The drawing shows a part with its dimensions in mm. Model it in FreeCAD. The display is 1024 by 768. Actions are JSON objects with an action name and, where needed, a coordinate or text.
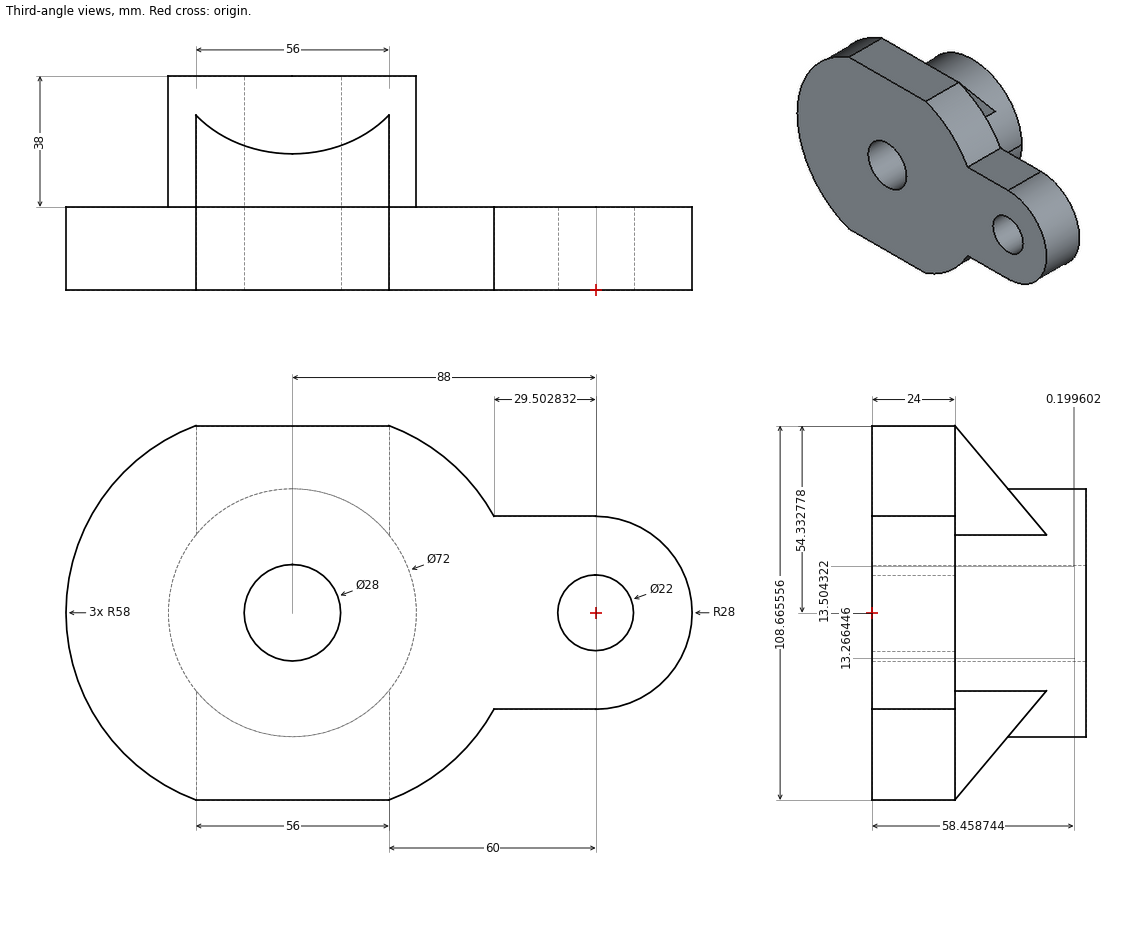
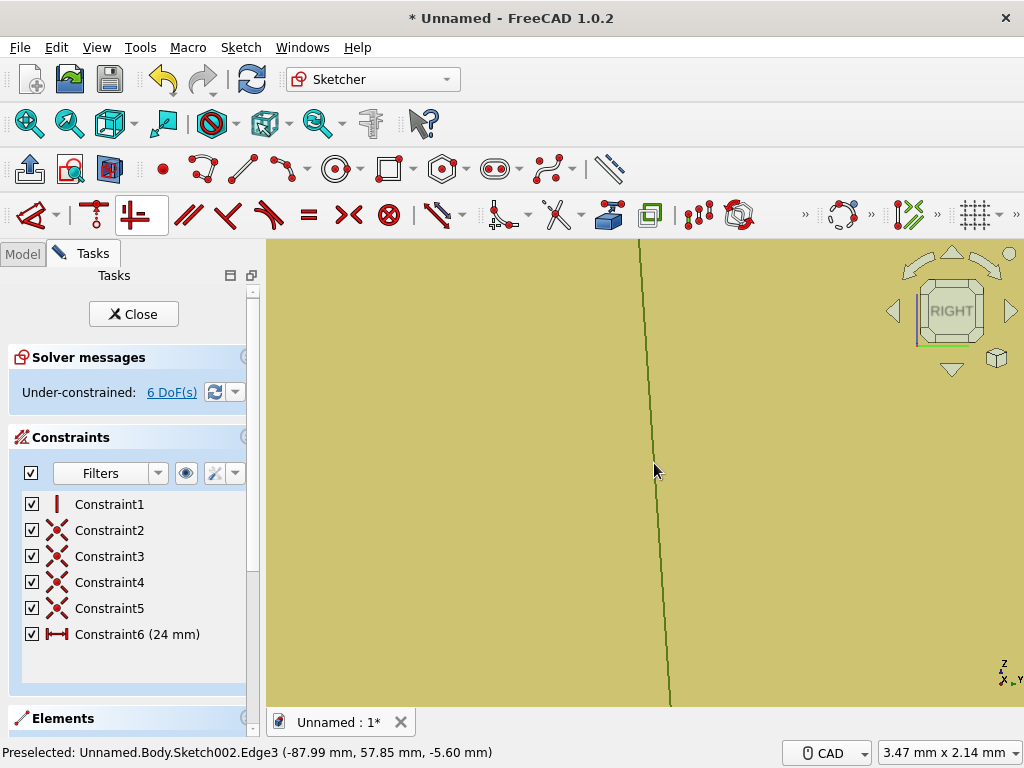
{"action": "left_click", "coordinate": [58, 216]}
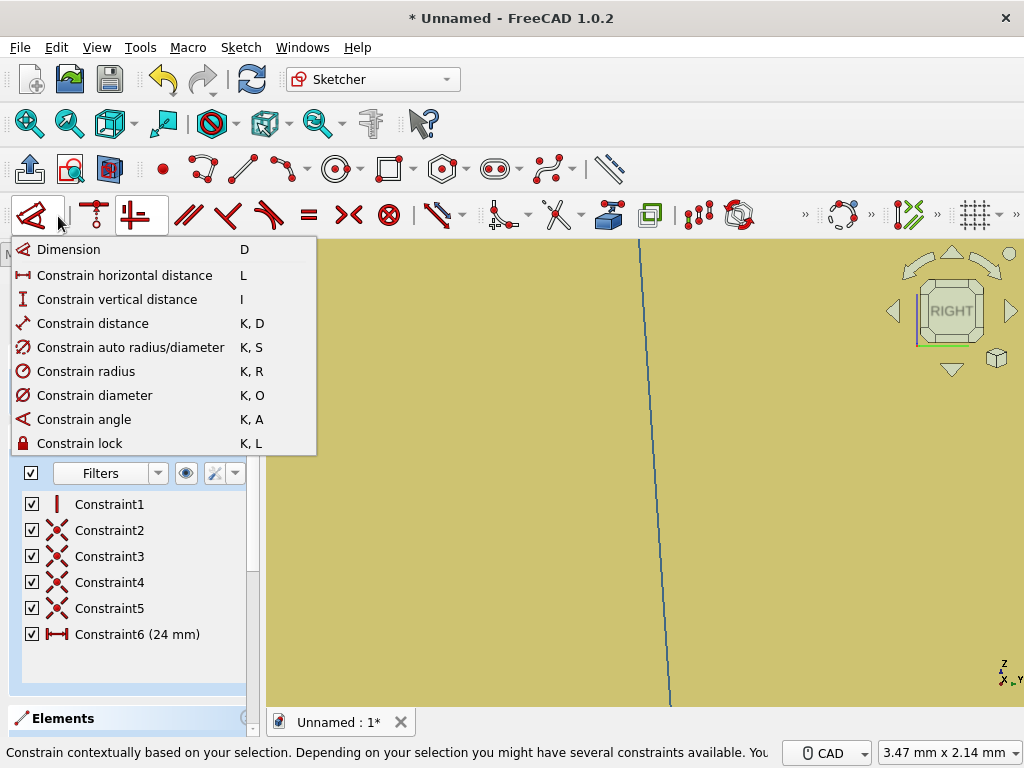
{"action": "left_click", "coordinate": [164, 275]}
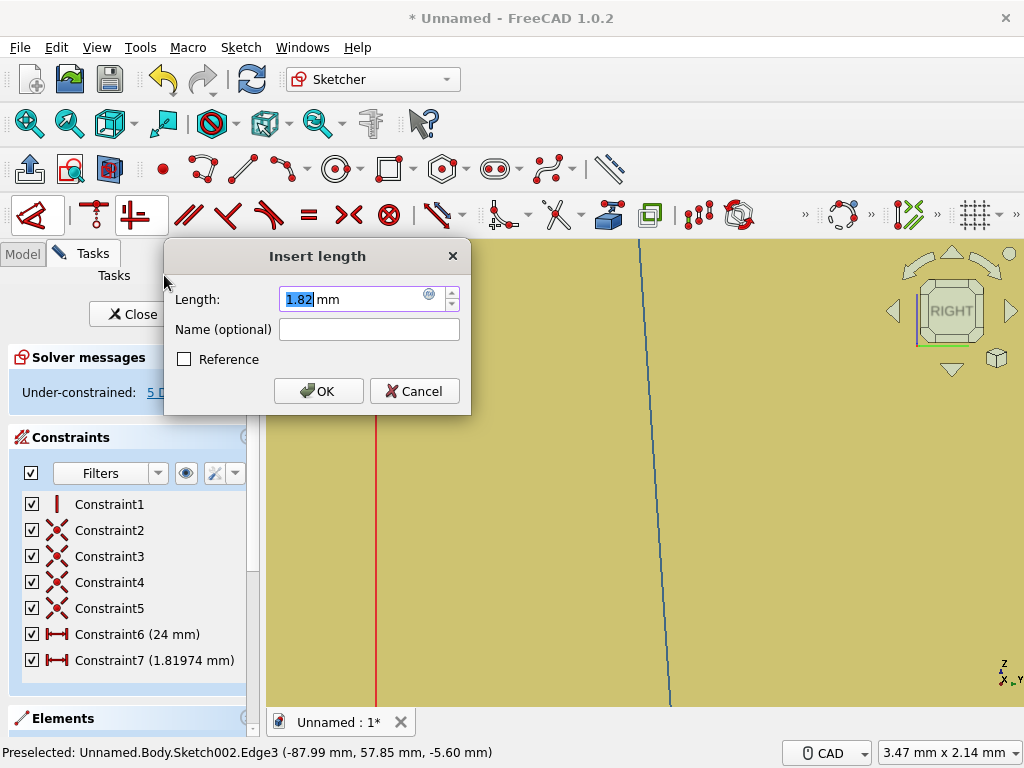
{"action": "type", "text": "0.199602"}
{"action": "key", "text": "Return"}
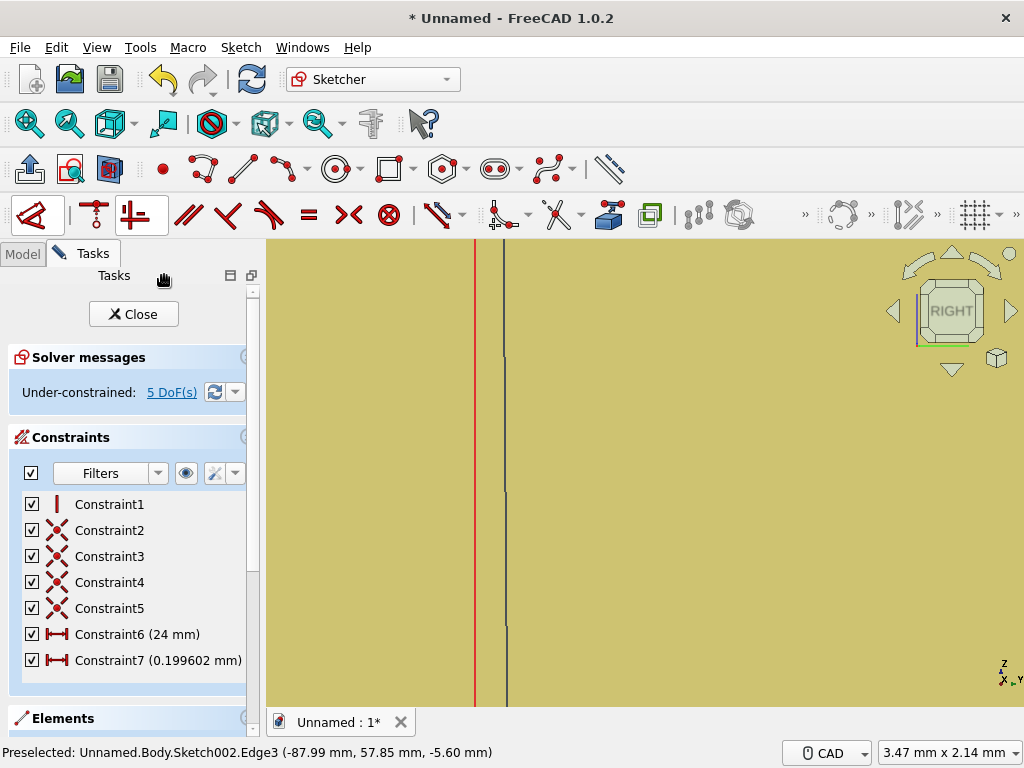
{"action": "scroll", "coordinate": [576, 473], "scroll_direction": "down", "scroll_amount": 15}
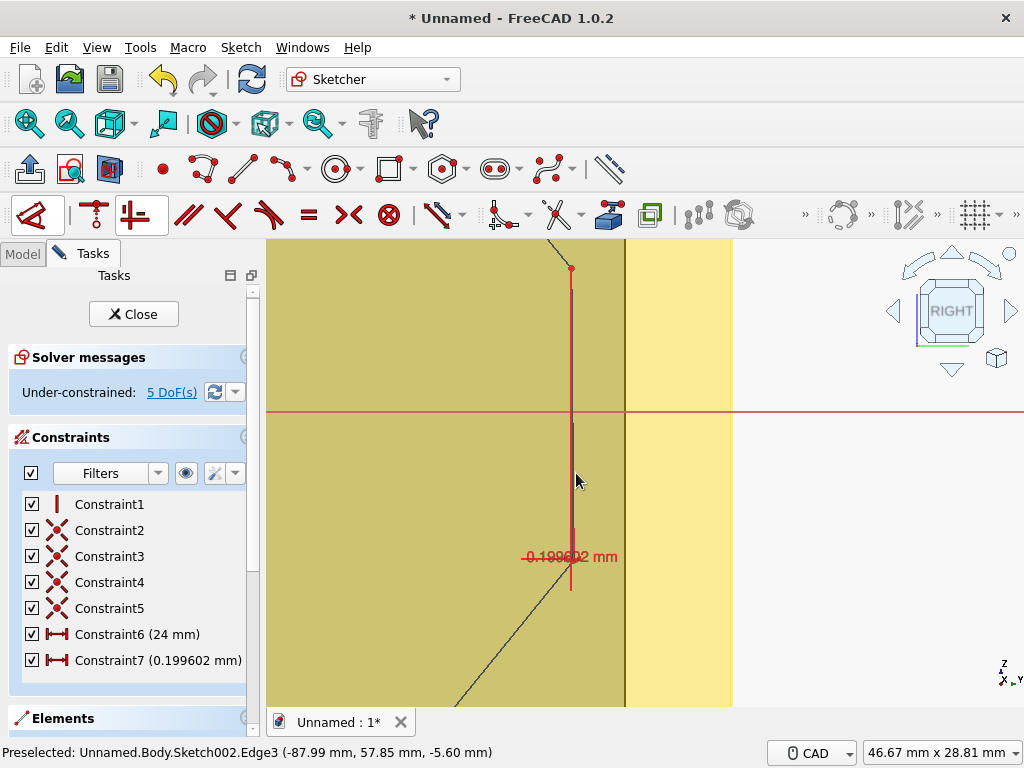
{"action": "scroll", "coordinate": [677, 493], "scroll_direction": "down", "scroll_amount": 7}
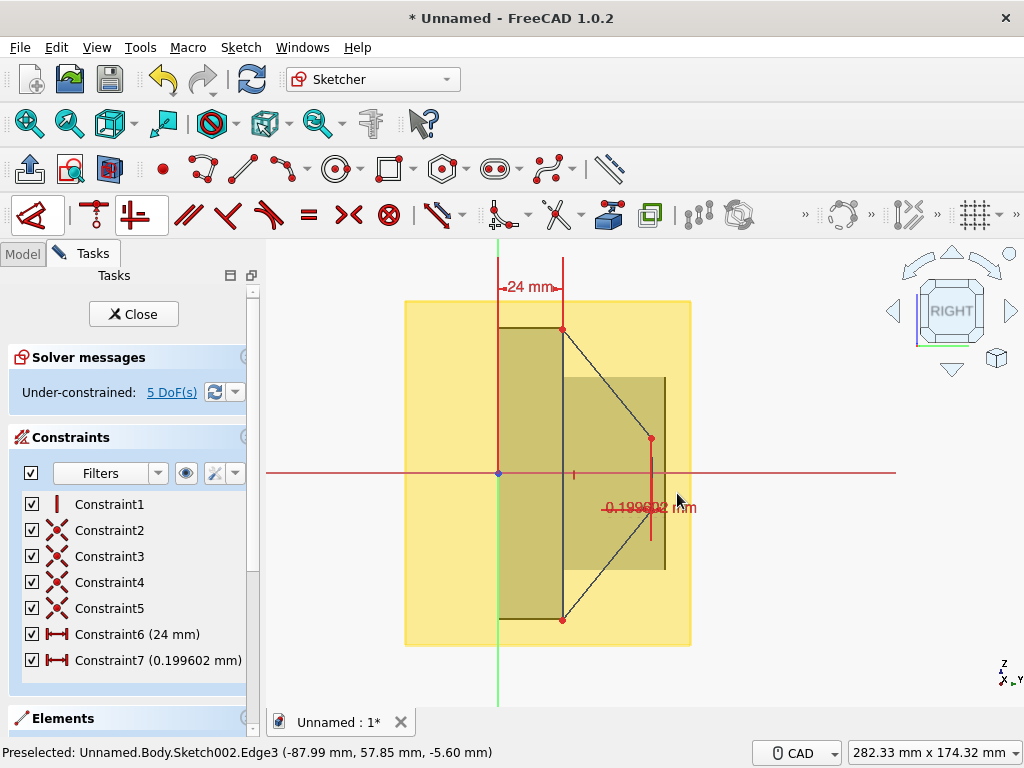
{"action": "left_click", "coordinate": [563, 417]}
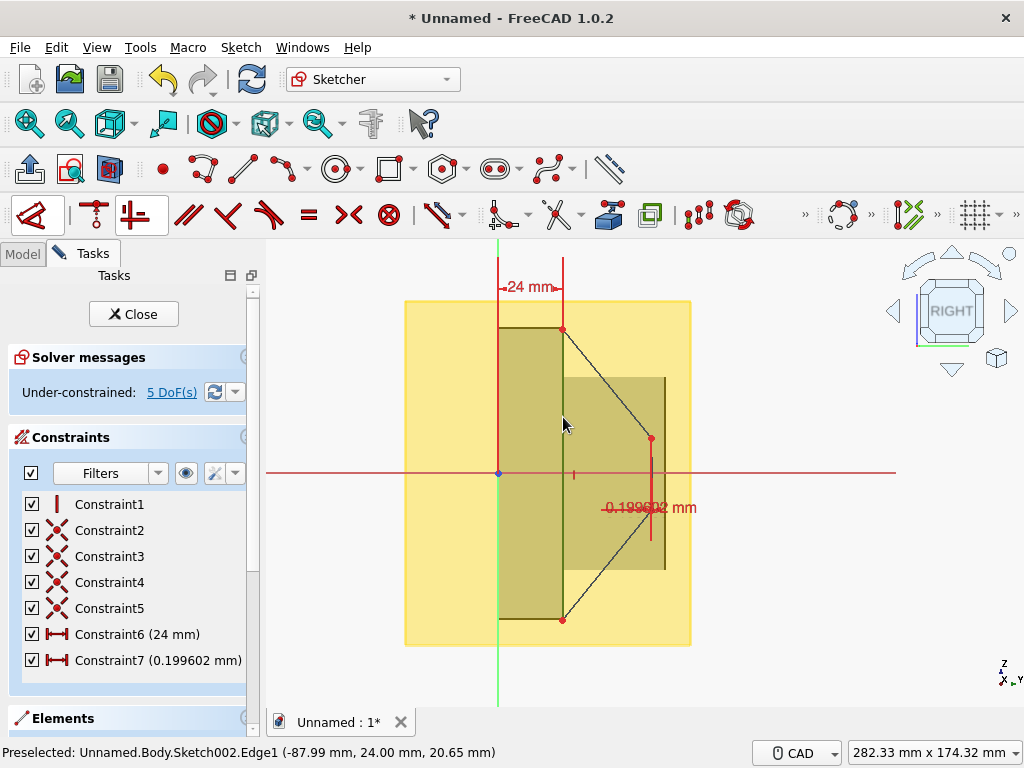
{"action": "left_click", "coordinate": [58, 216]}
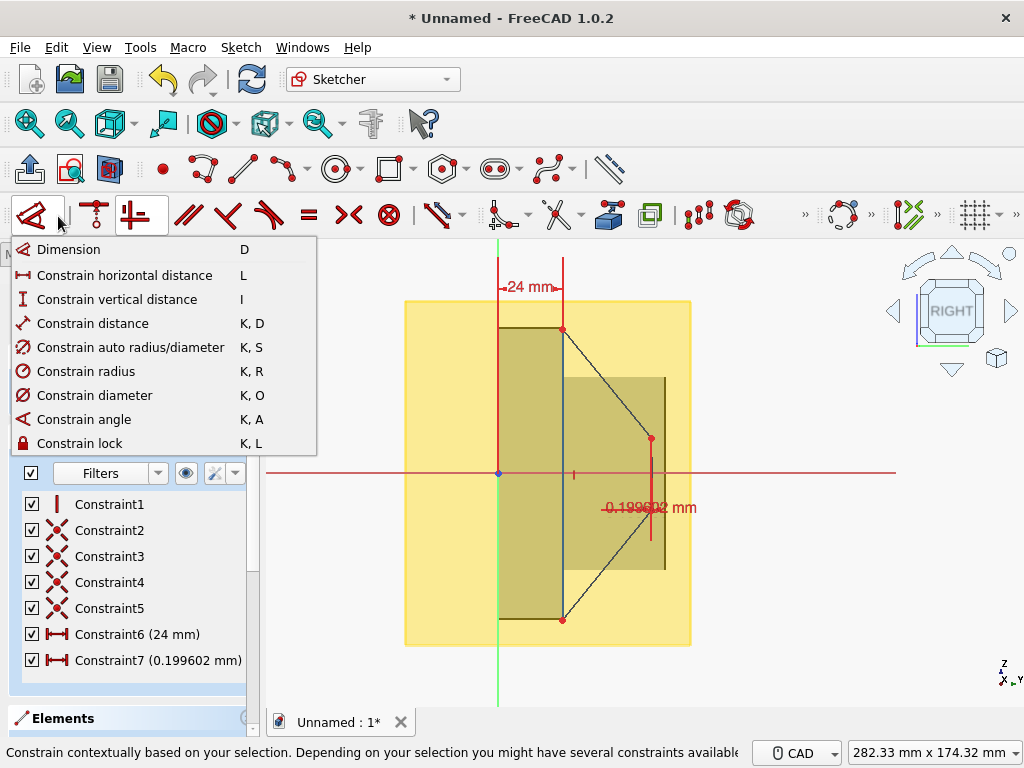
{"action": "left_click", "coordinate": [164, 299]}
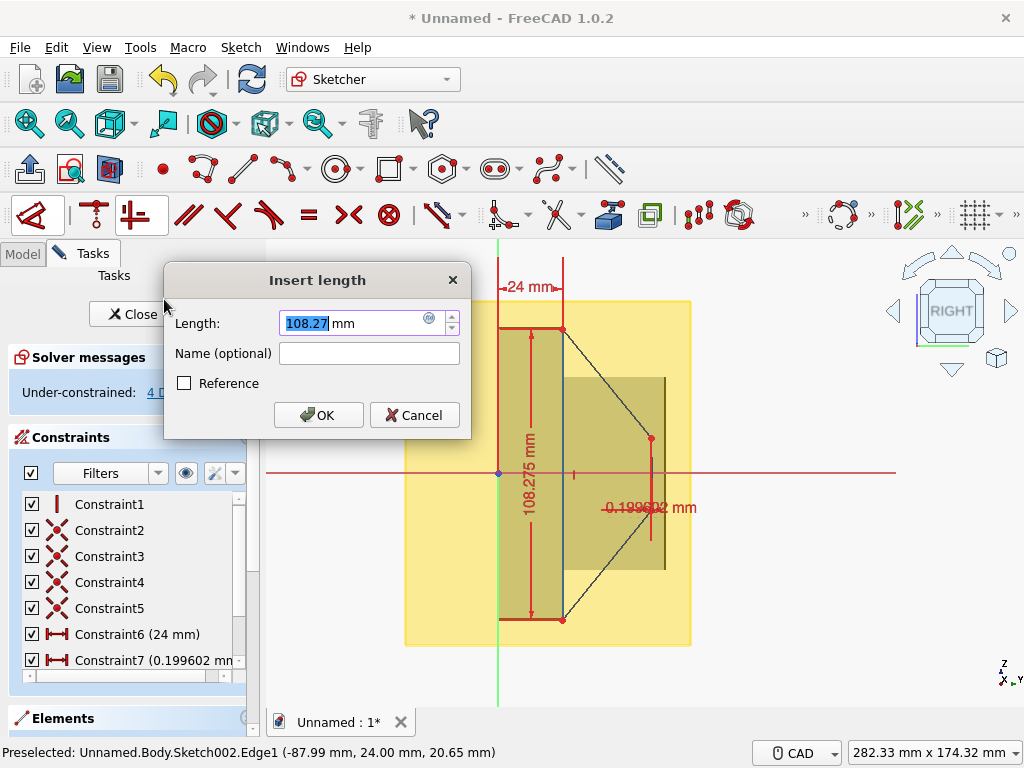
{"action": "type", "text": "108.665556"}
{"action": "key", "text": "Return"}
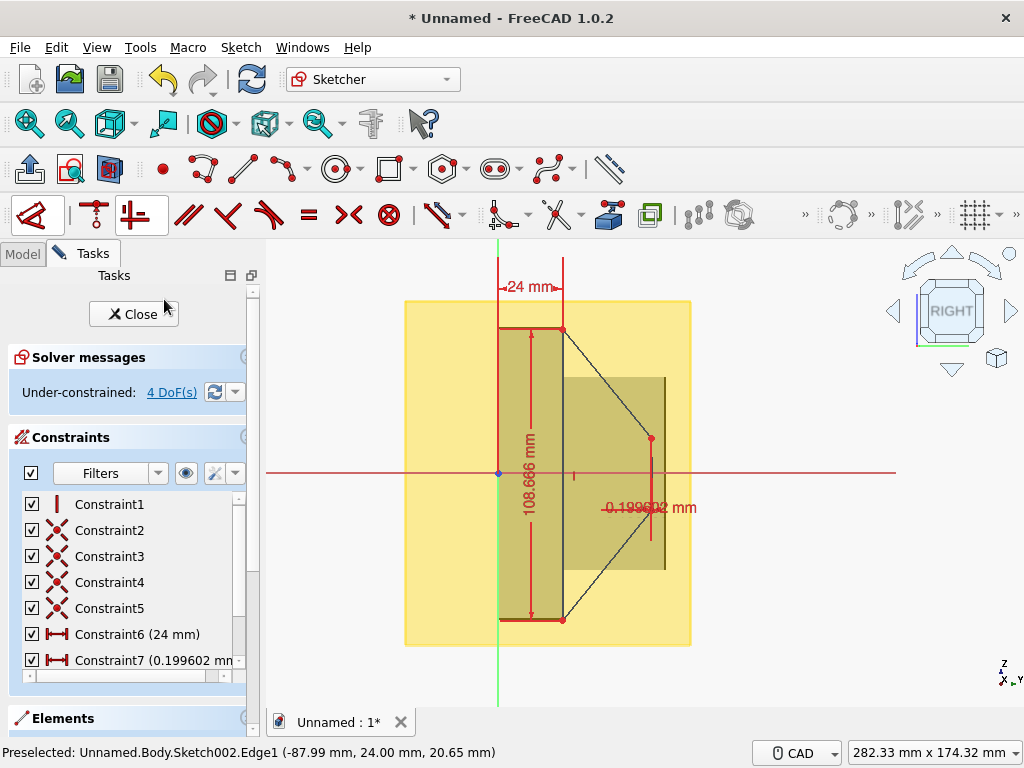
{"action": "left_click", "coordinate": [563, 329]}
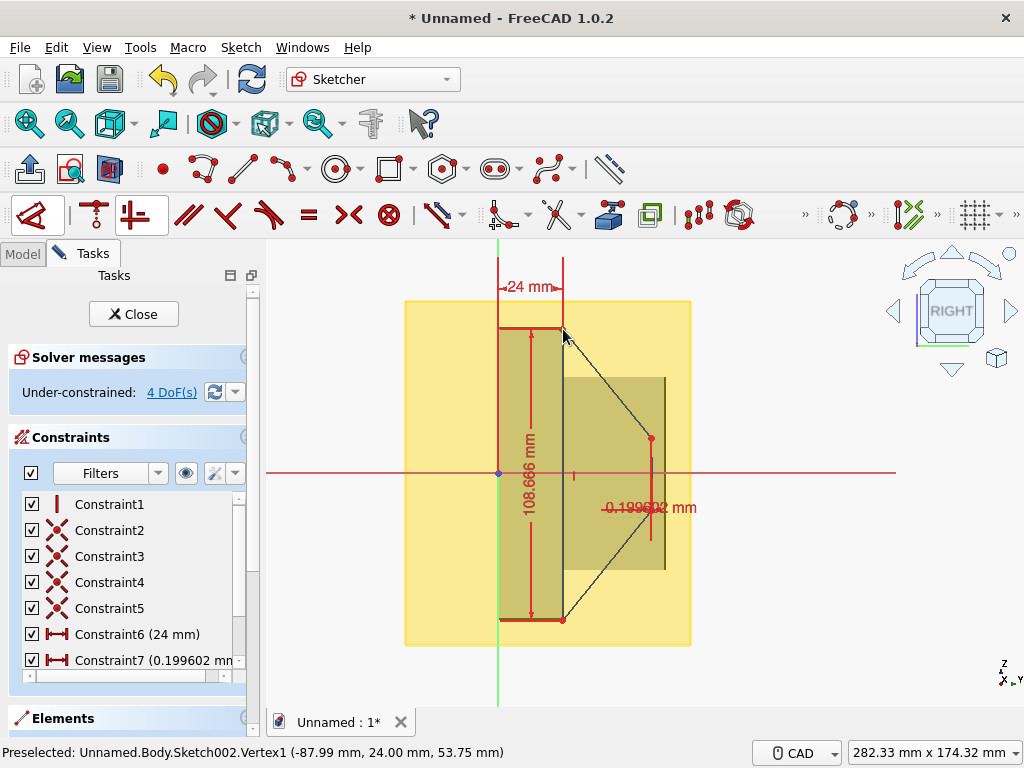
{"action": "left_click", "coordinate": [58, 216]}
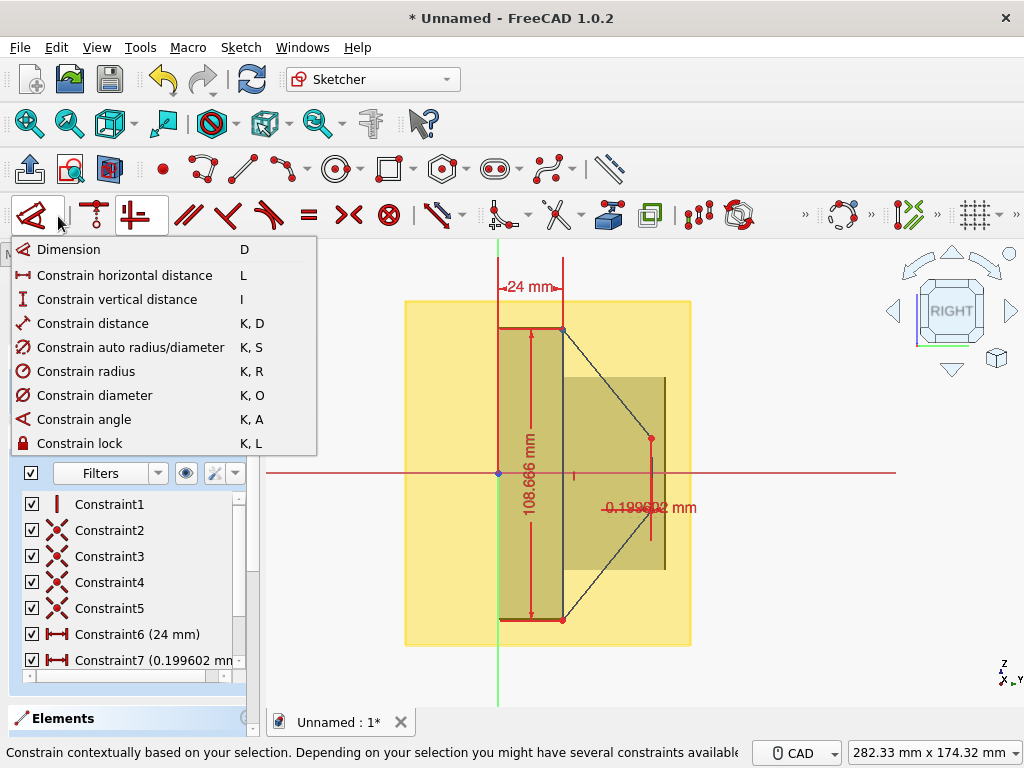
{"action": "left_click", "coordinate": [164, 299]}